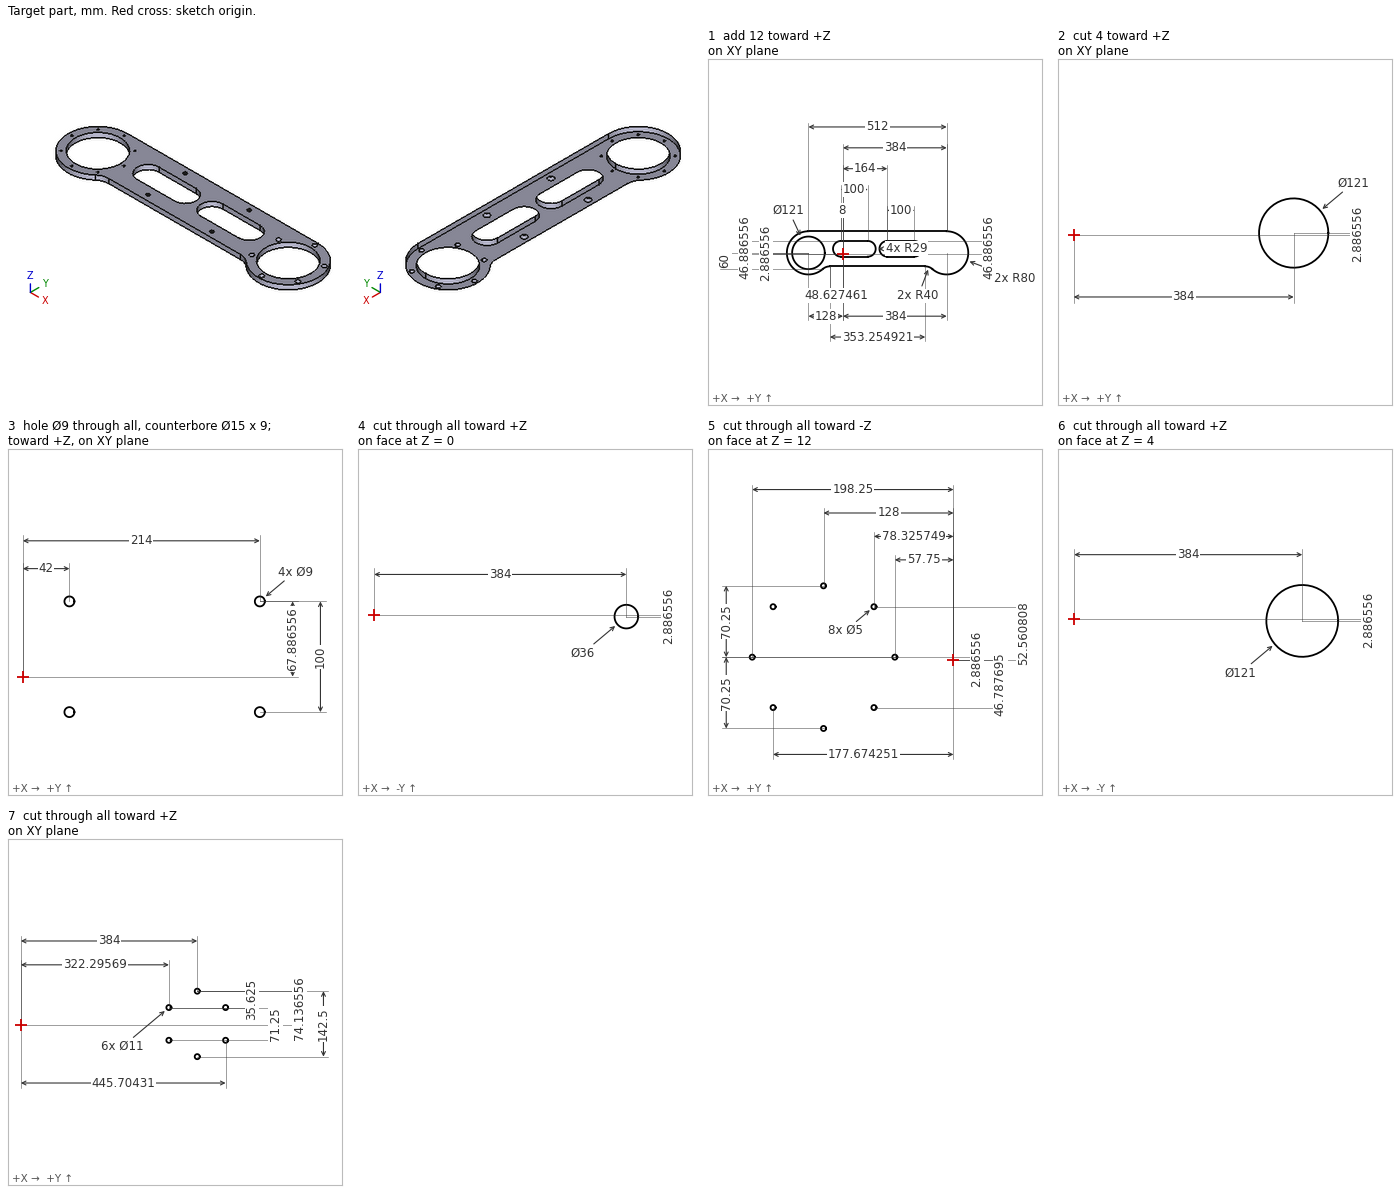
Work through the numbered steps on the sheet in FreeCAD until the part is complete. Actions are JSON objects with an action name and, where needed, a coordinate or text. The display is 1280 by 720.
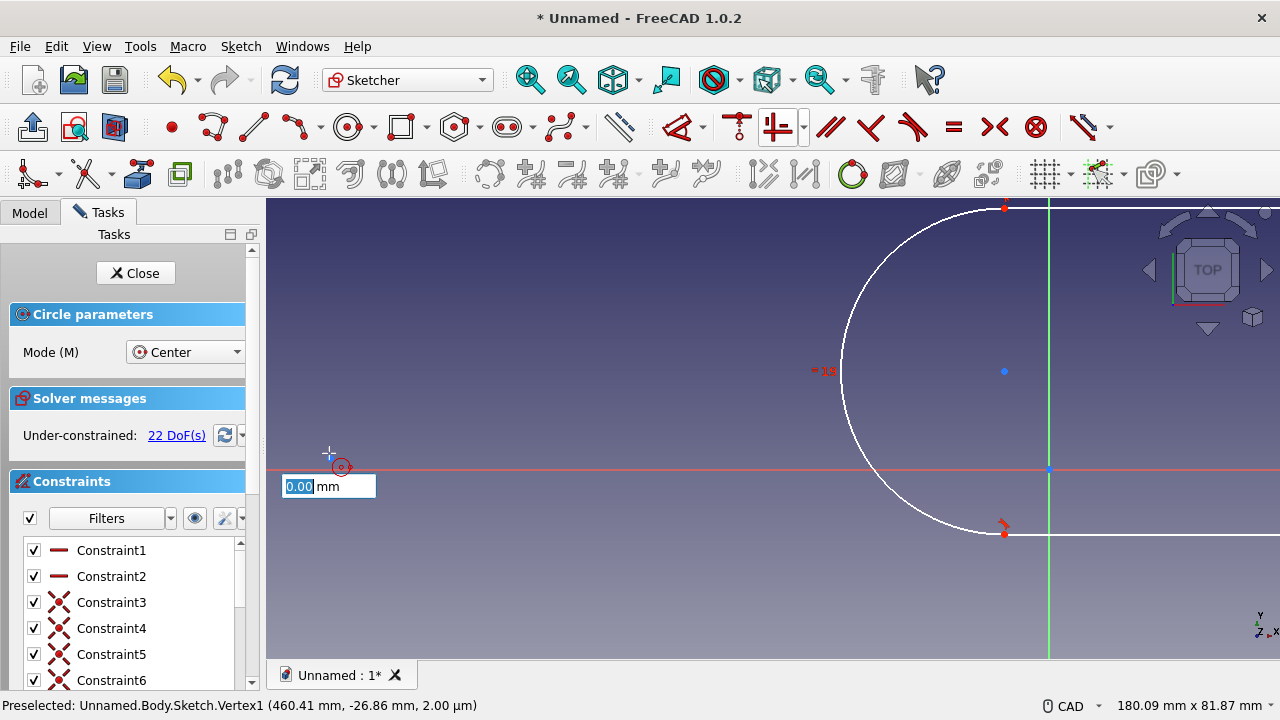
{"action": "scroll", "coordinate": [493, 434], "scroll_direction": "down", "scroll_amount": 9}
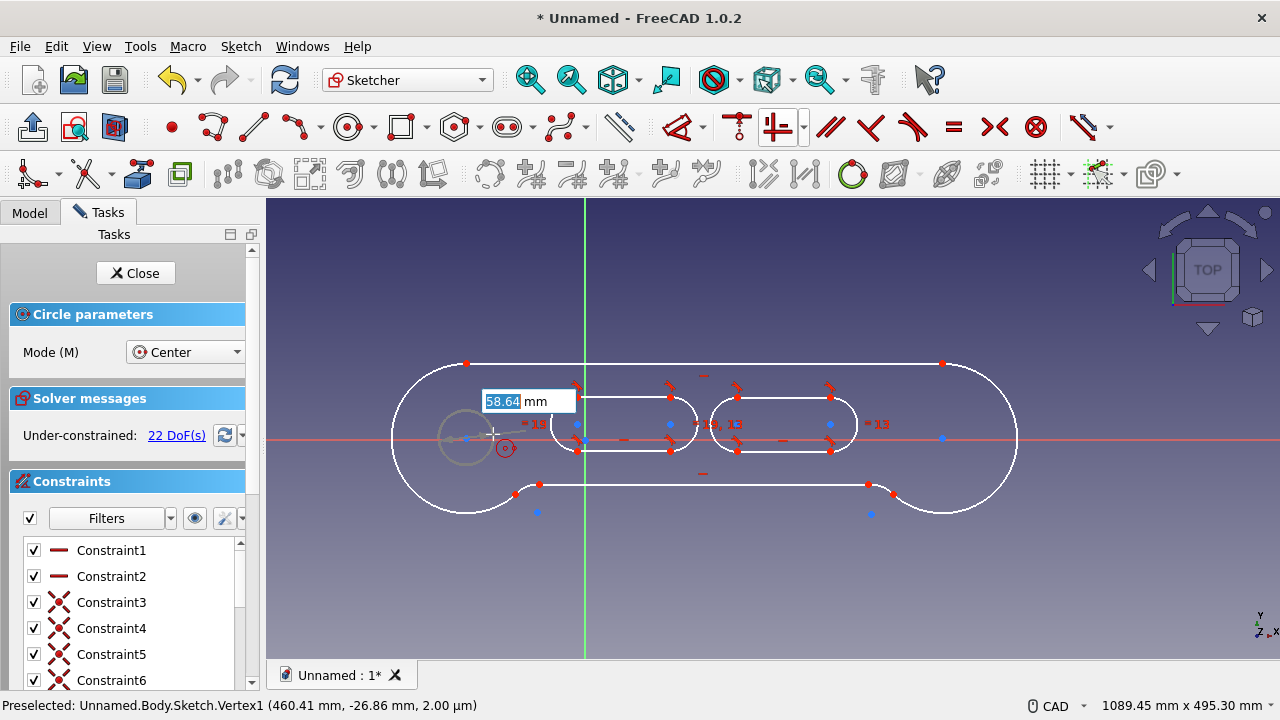
{"action": "left_click", "coordinate": [506, 398]}
{"action": "key", "text": "Escape"}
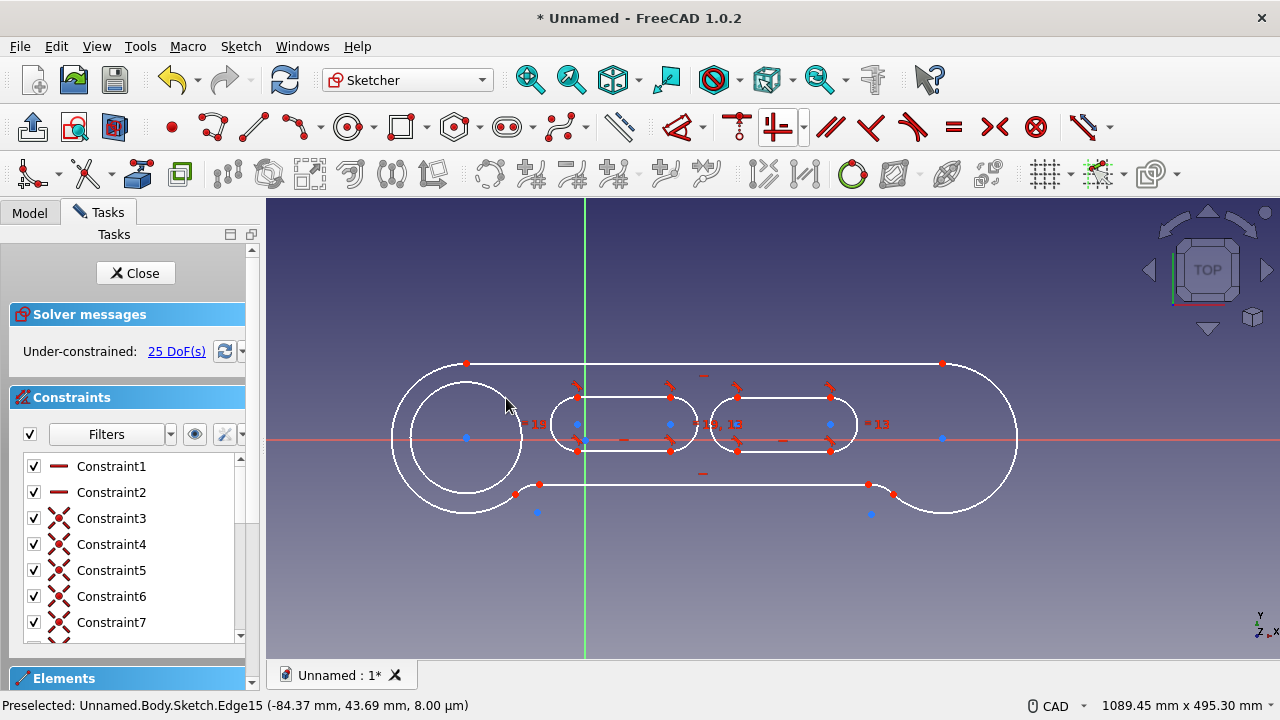
{"action": "left_click", "coordinate": [398, 408]}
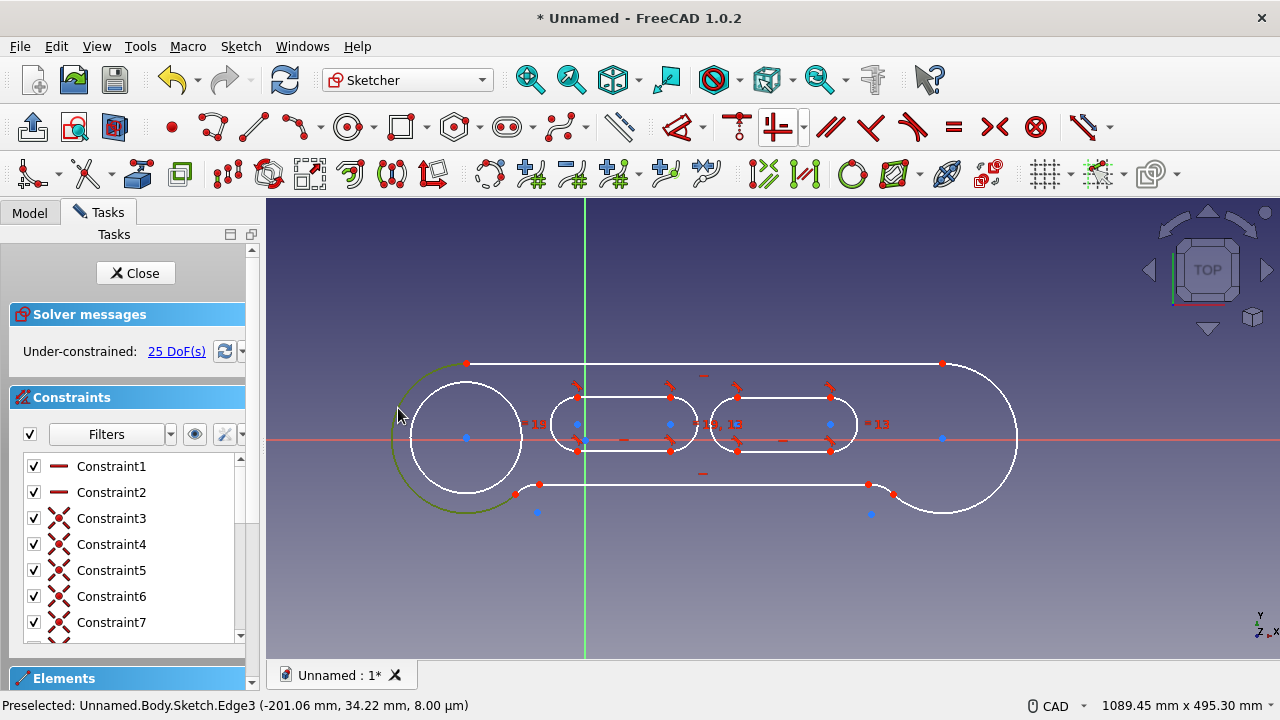
{"action": "left_click", "coordinate": [526, 487]}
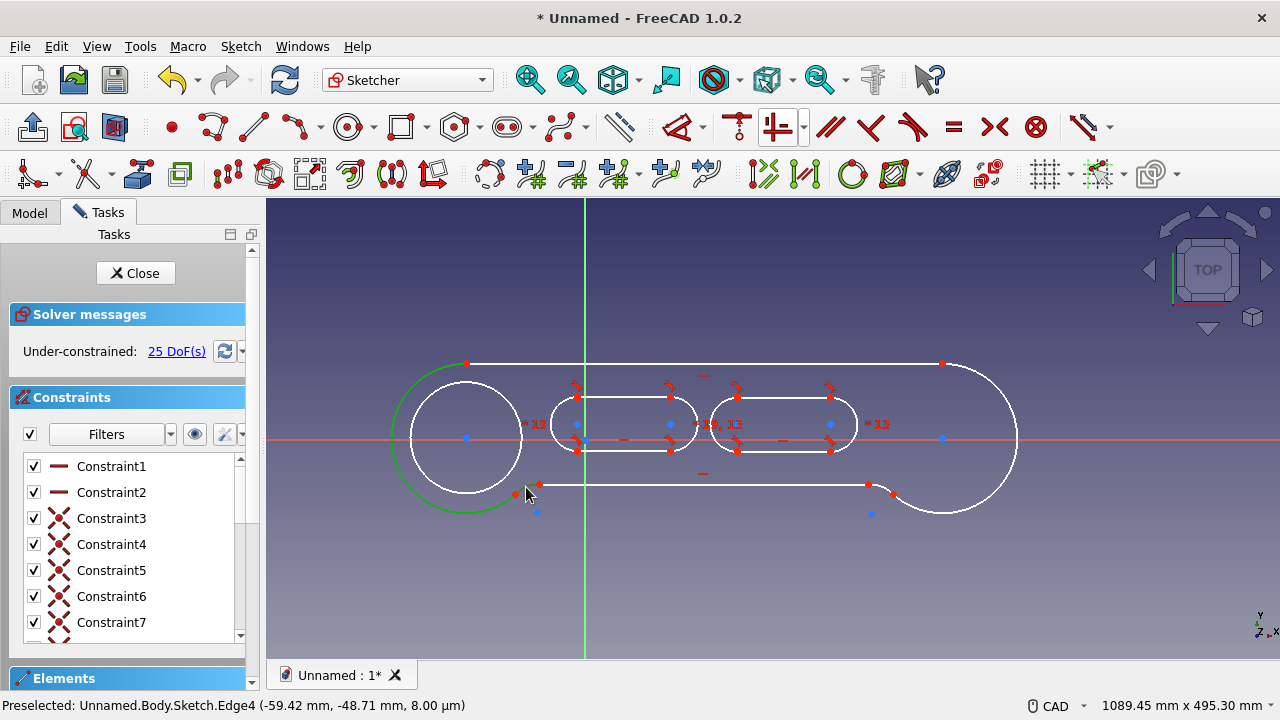
{"action": "left_click", "coordinate": [913, 128]}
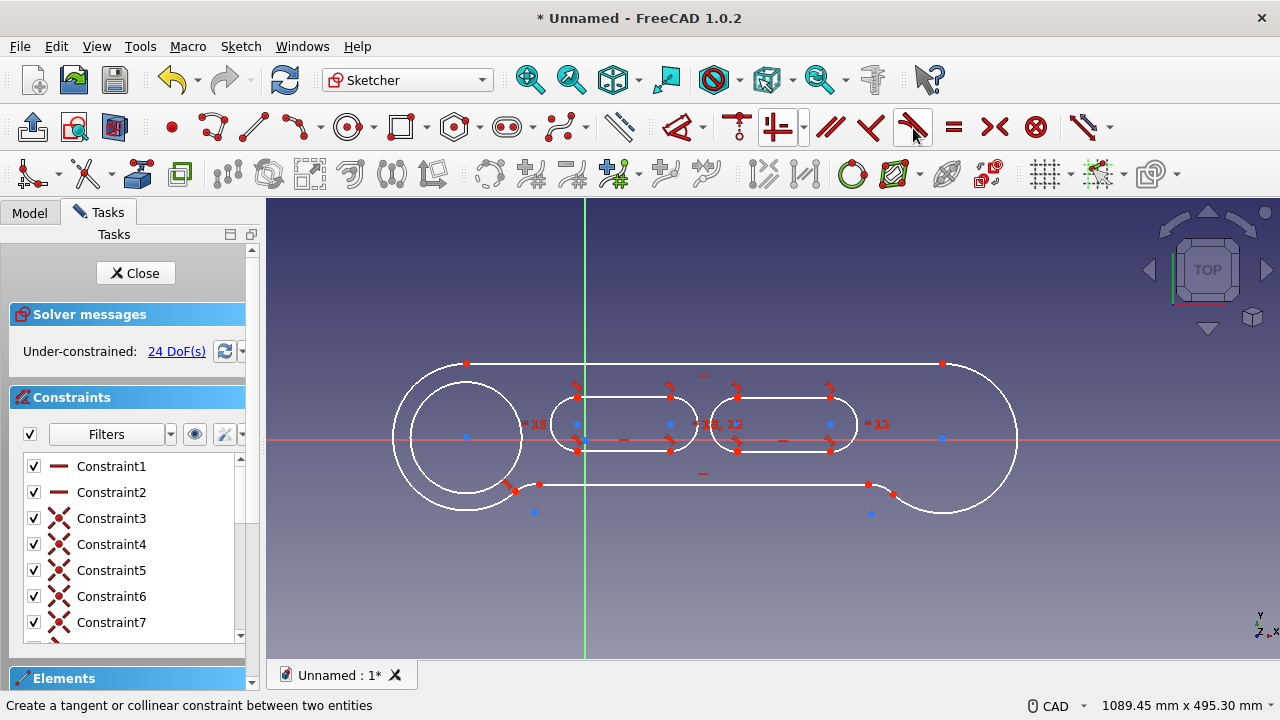
{"action": "left_click", "coordinate": [882, 487]}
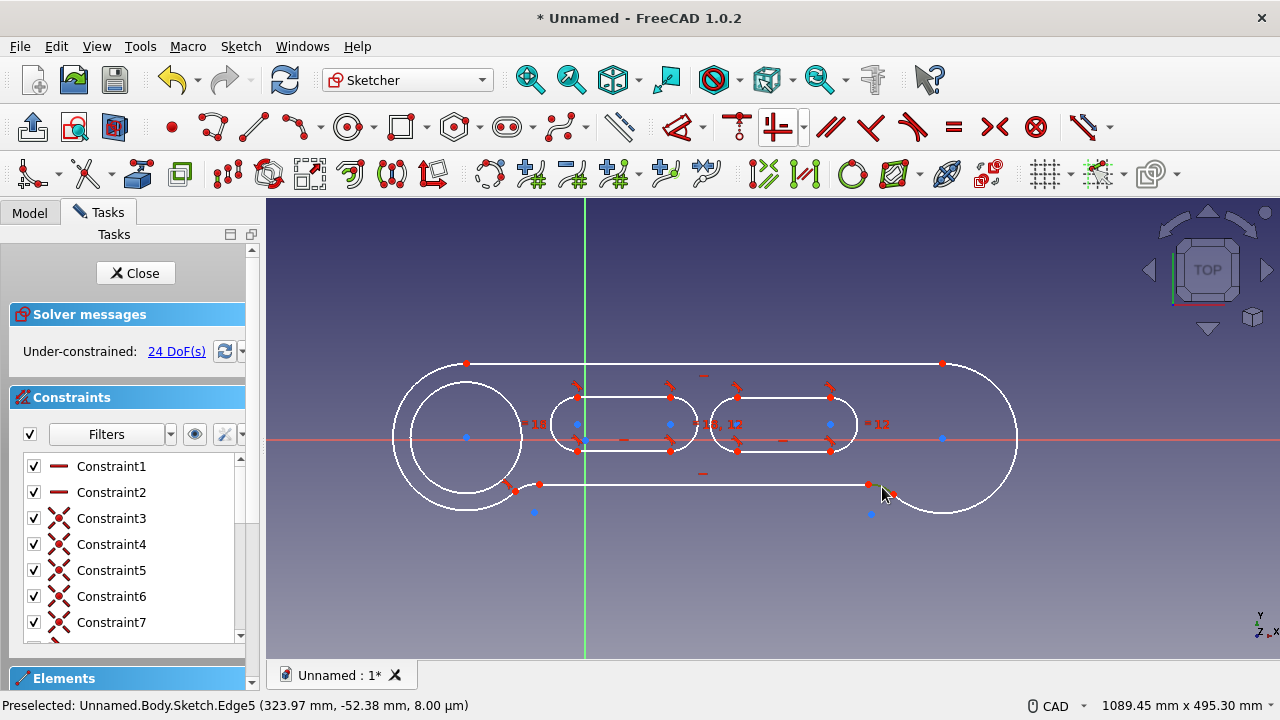
{"action": "left_click", "coordinate": [974, 506]}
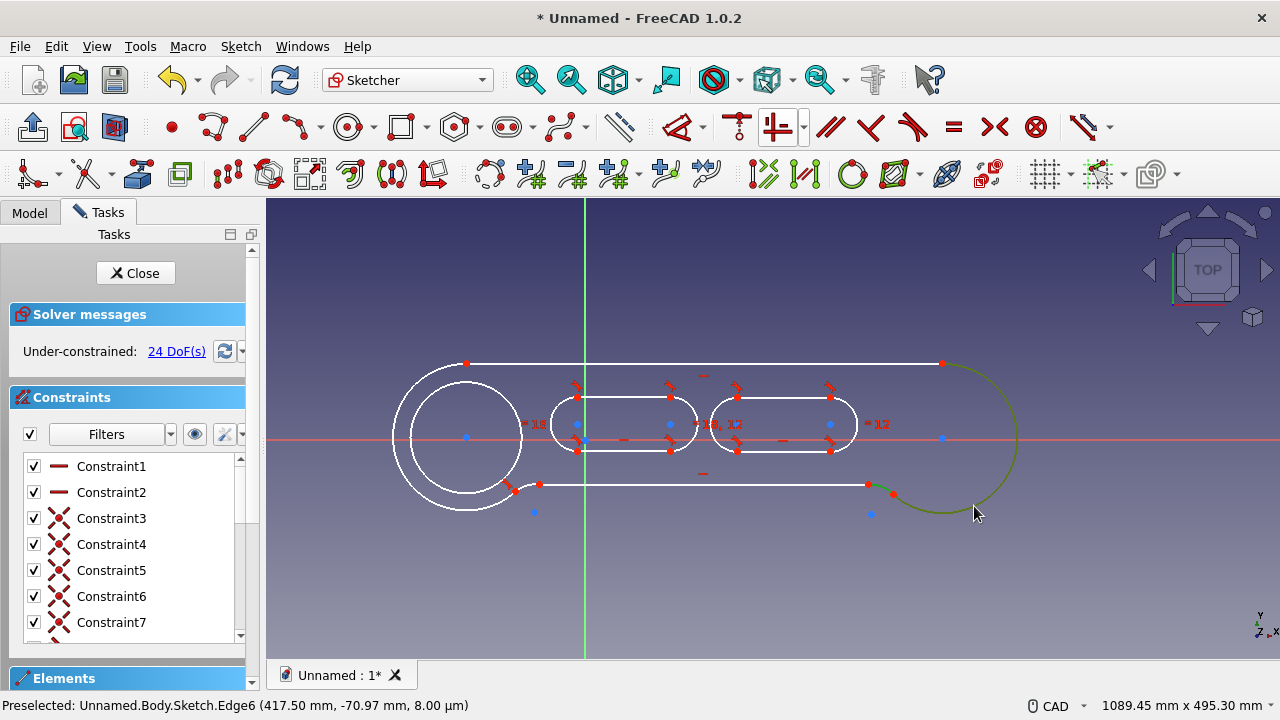
{"action": "left_click", "coordinate": [913, 128]}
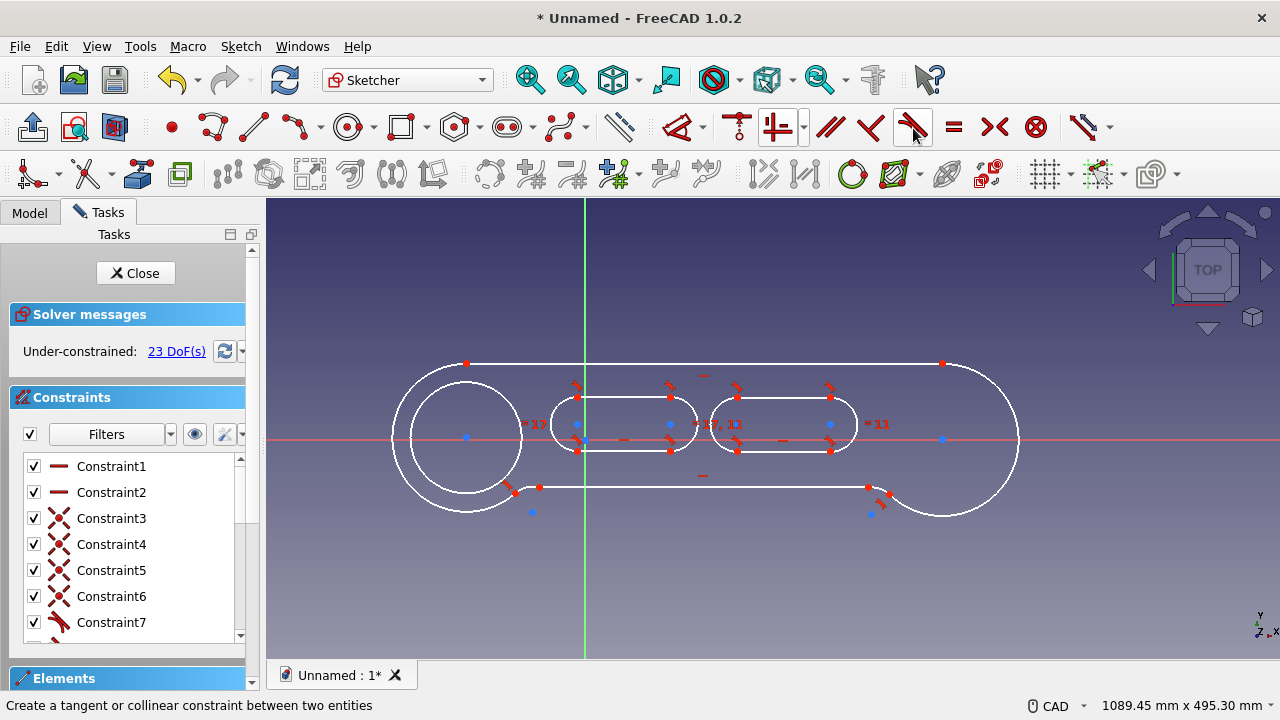
{"action": "left_click", "coordinate": [505, 398]}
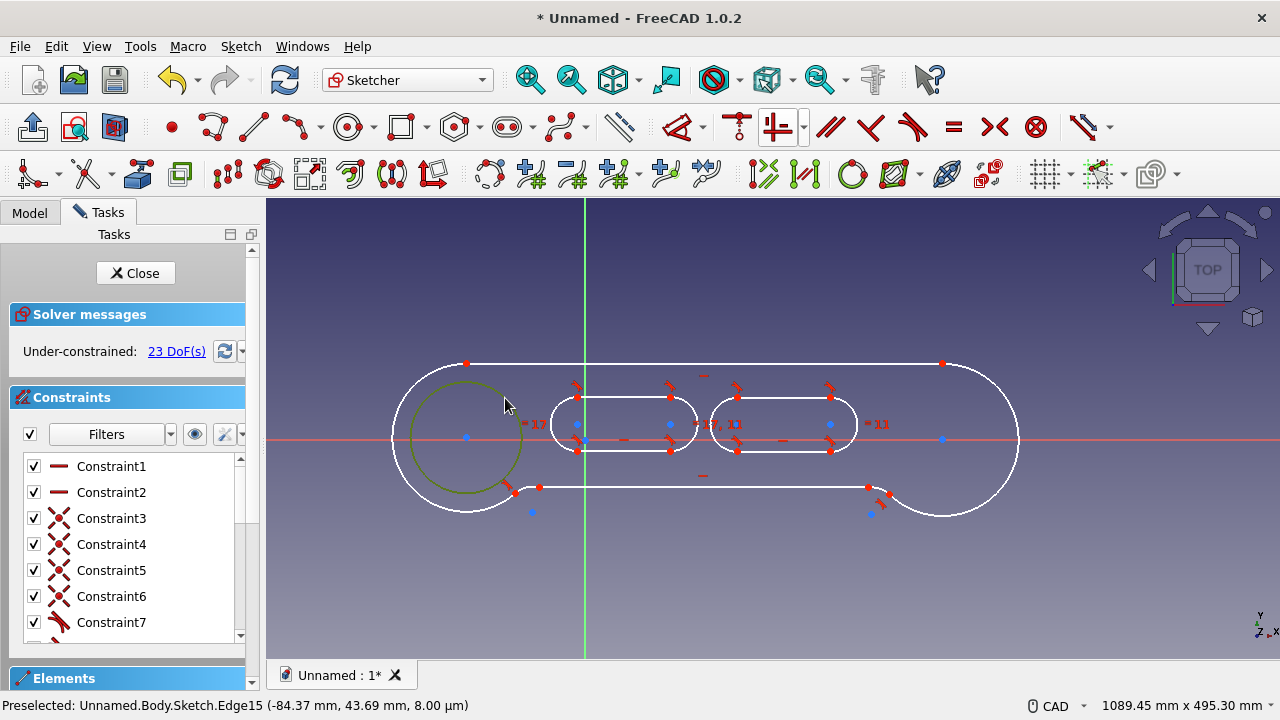
{"action": "left_click", "coordinate": [399, 408]}